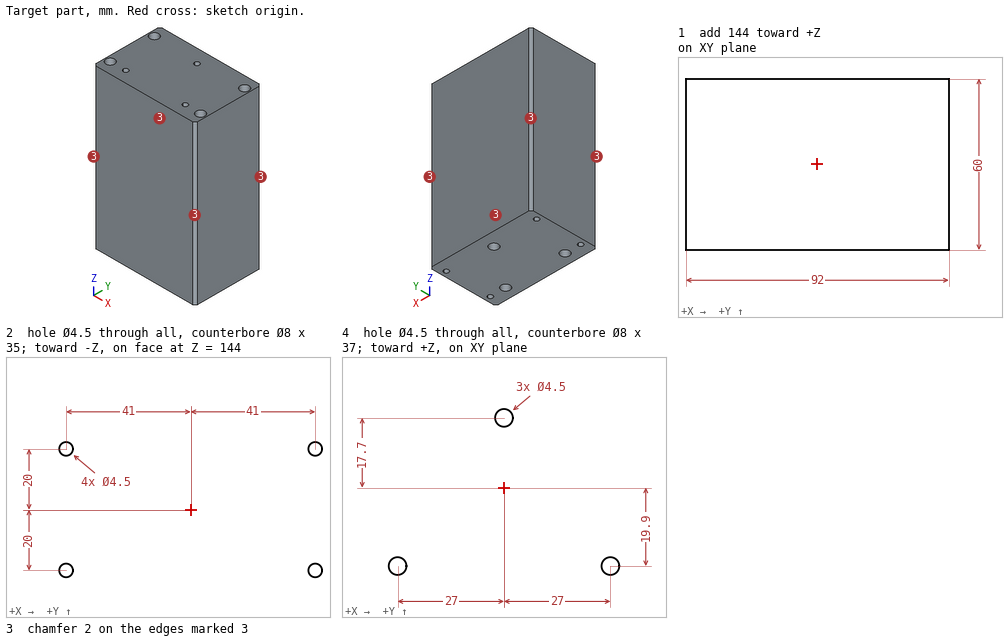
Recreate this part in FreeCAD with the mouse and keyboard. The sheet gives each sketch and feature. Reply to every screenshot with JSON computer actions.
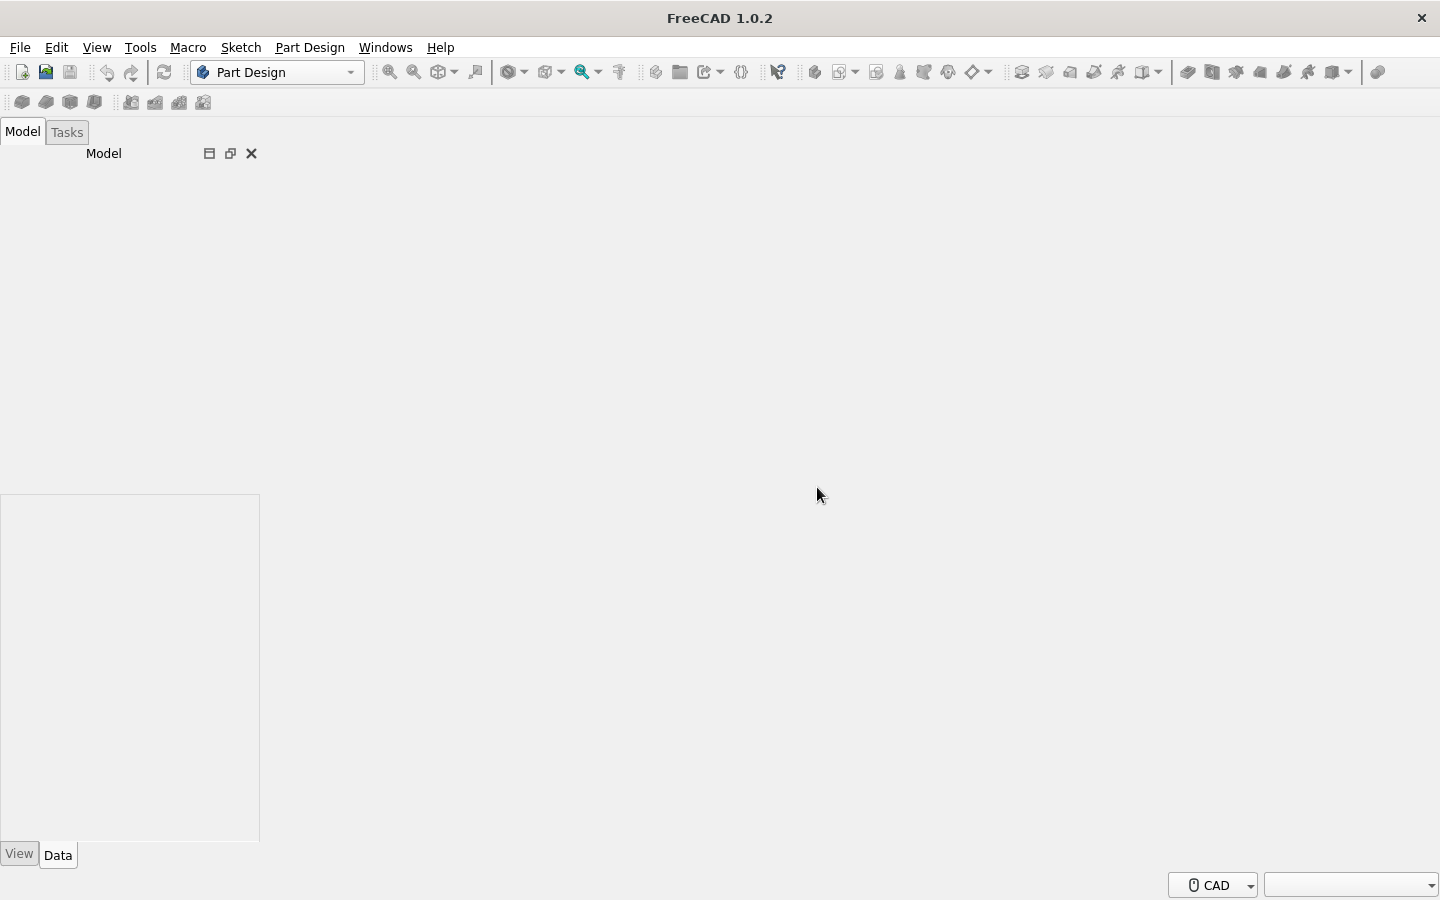
{"action": "left_click", "coordinate": [22, 72]}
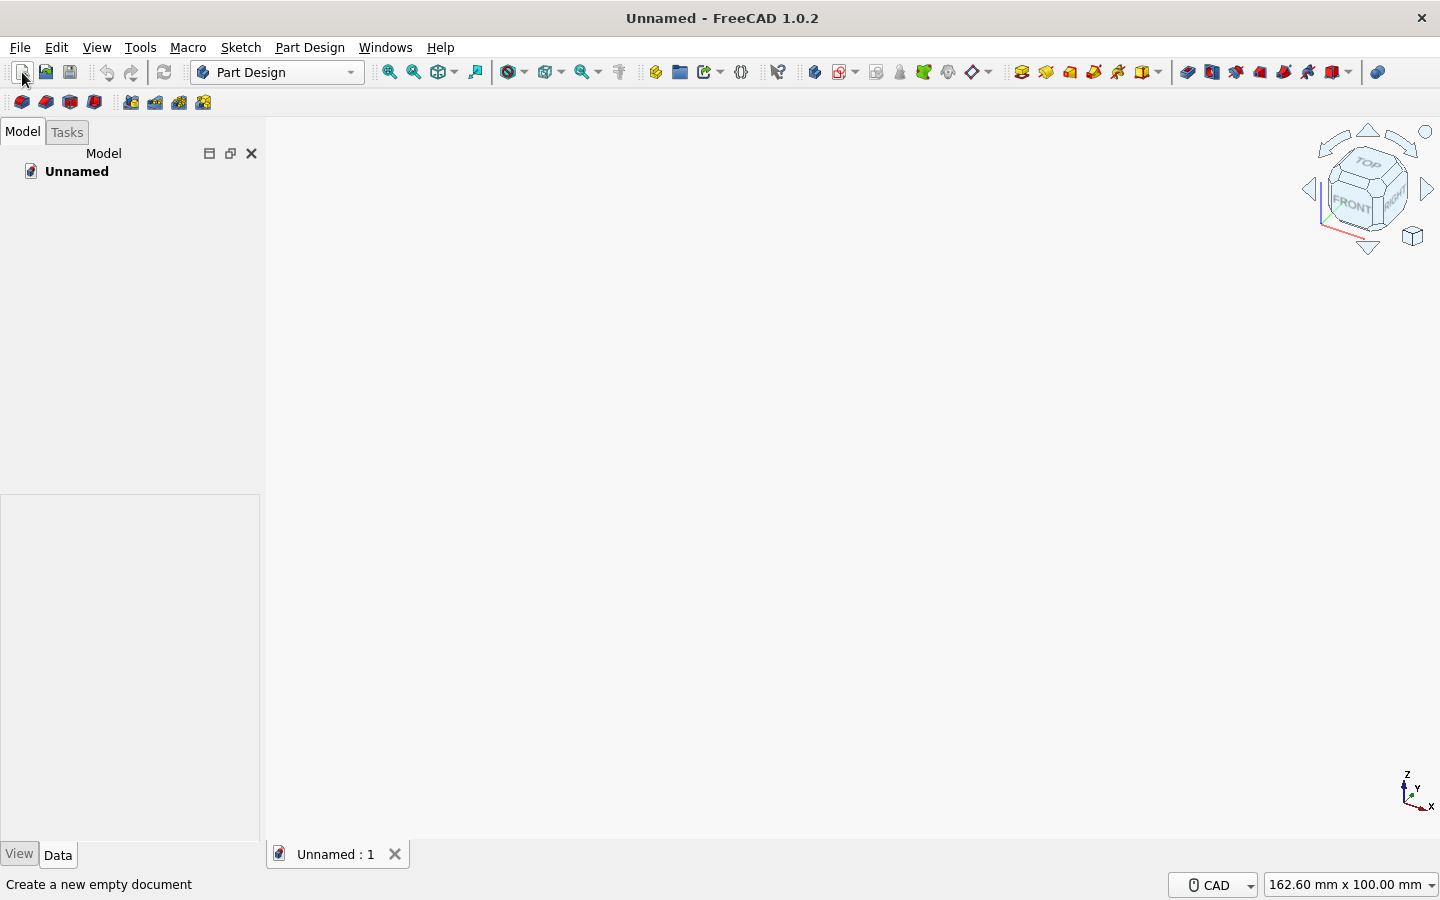
{"action": "left_click", "coordinate": [840, 72]}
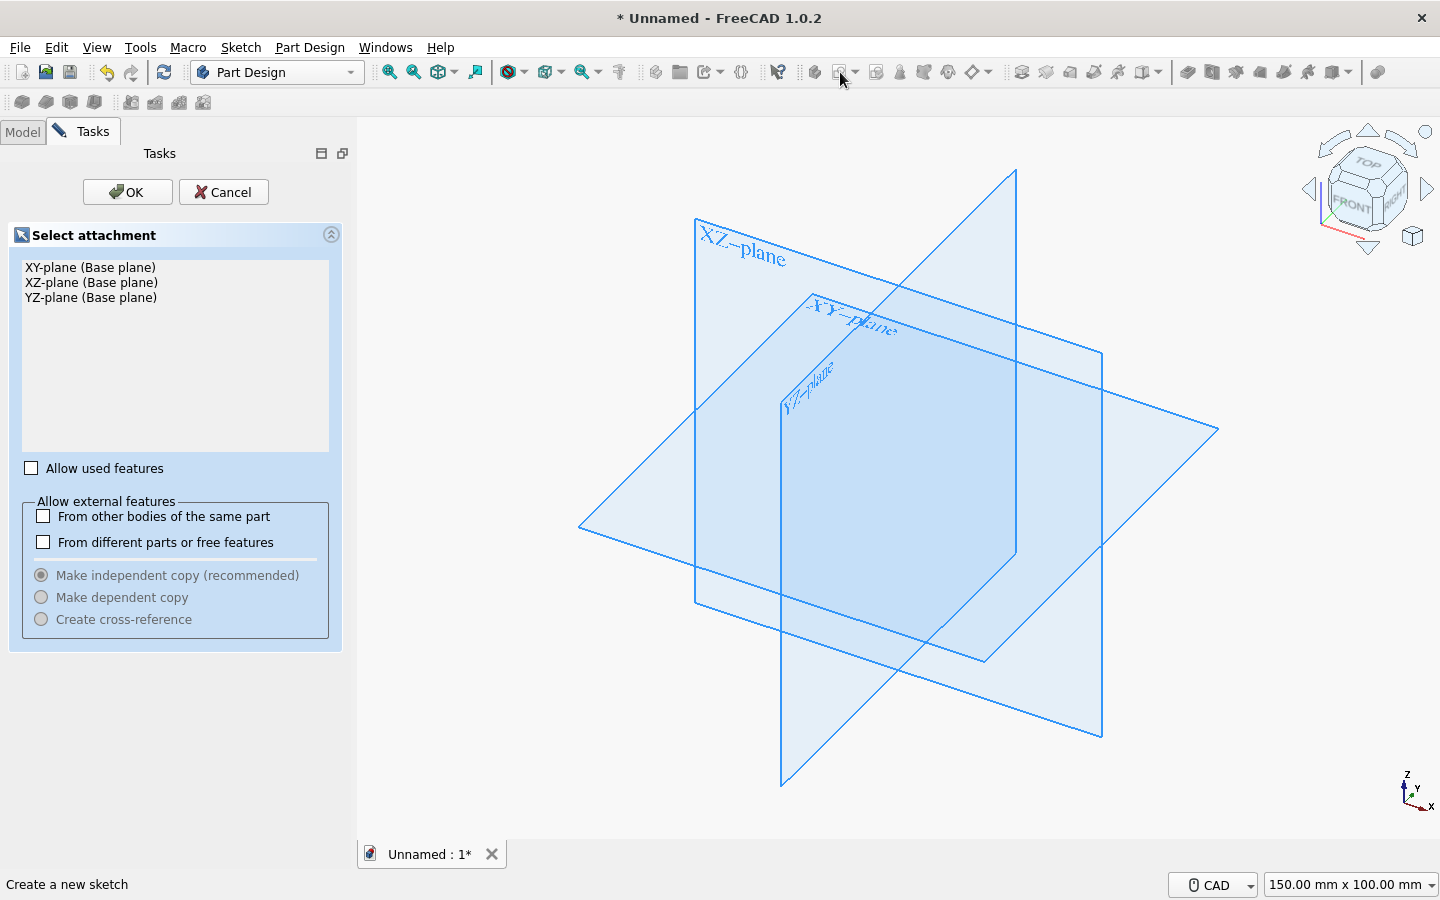
{"action": "left_click", "coordinate": [82, 268]}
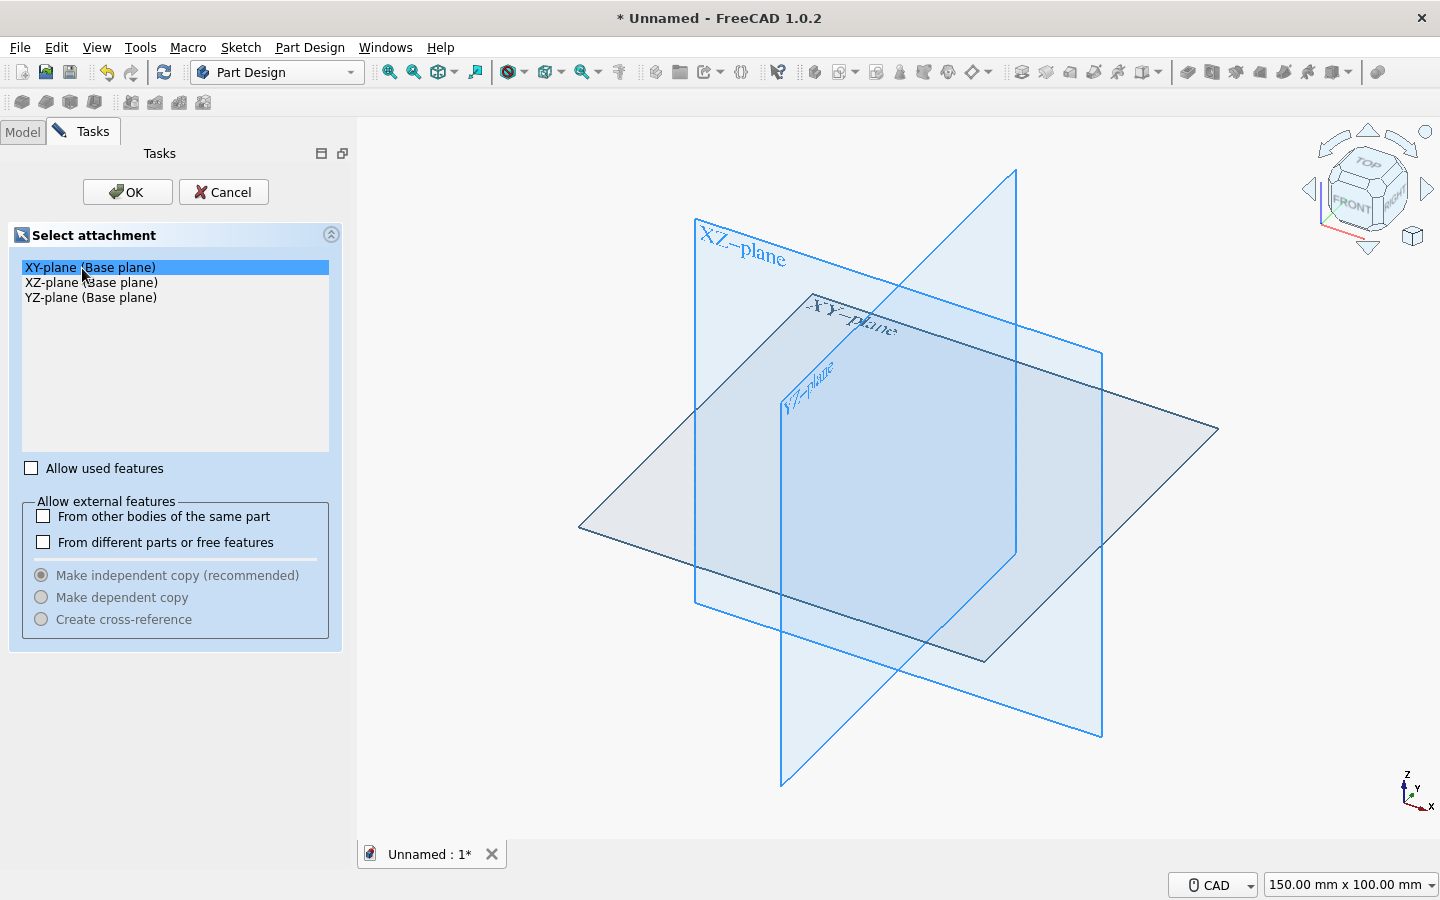
{"action": "left_click", "coordinate": [128, 192]}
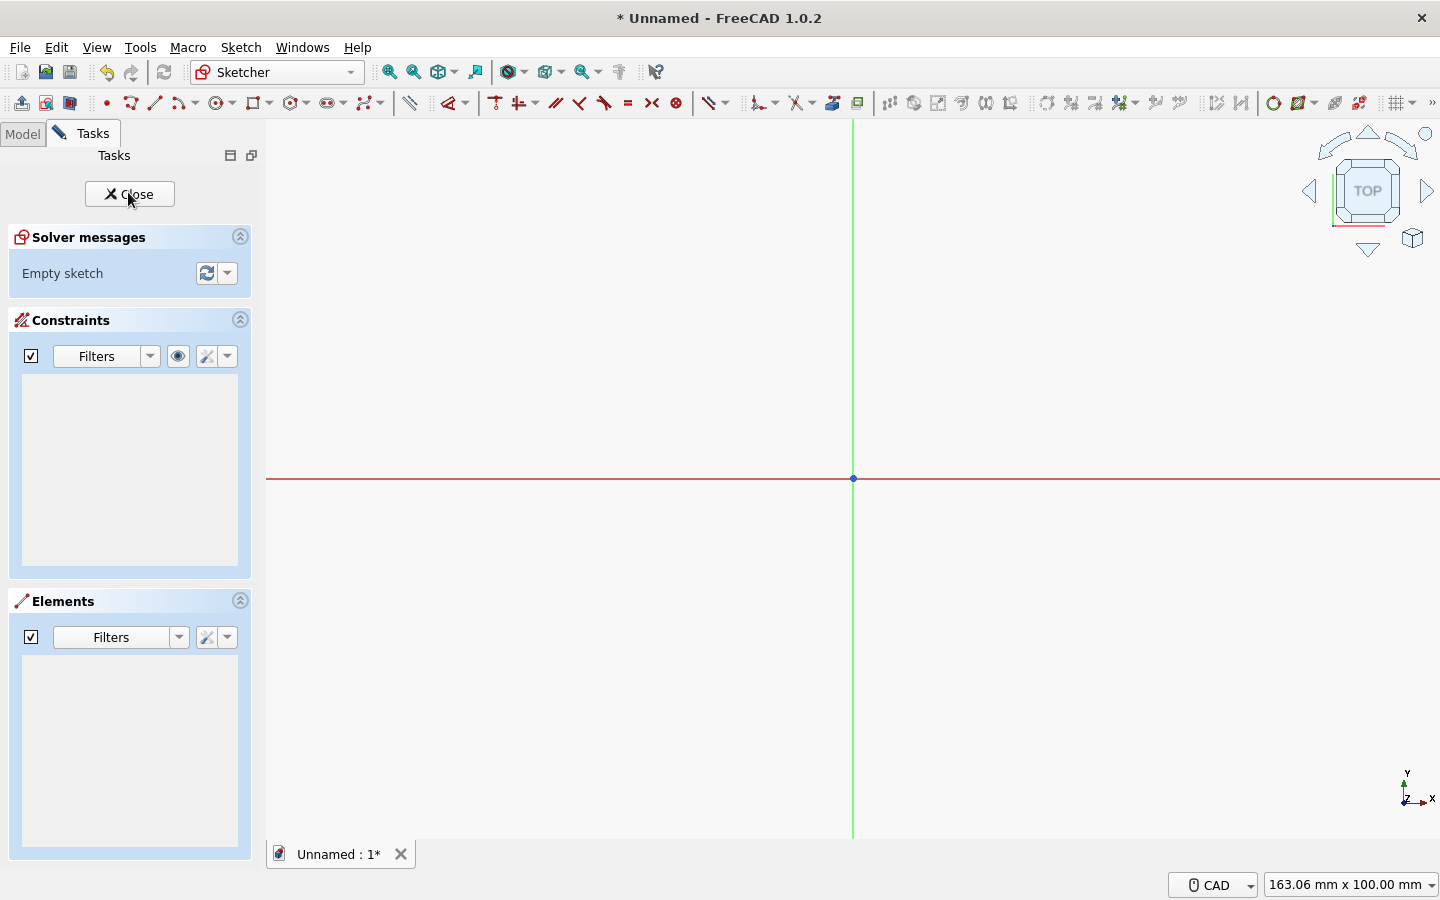
{"action": "left_click", "coordinate": [272, 104]}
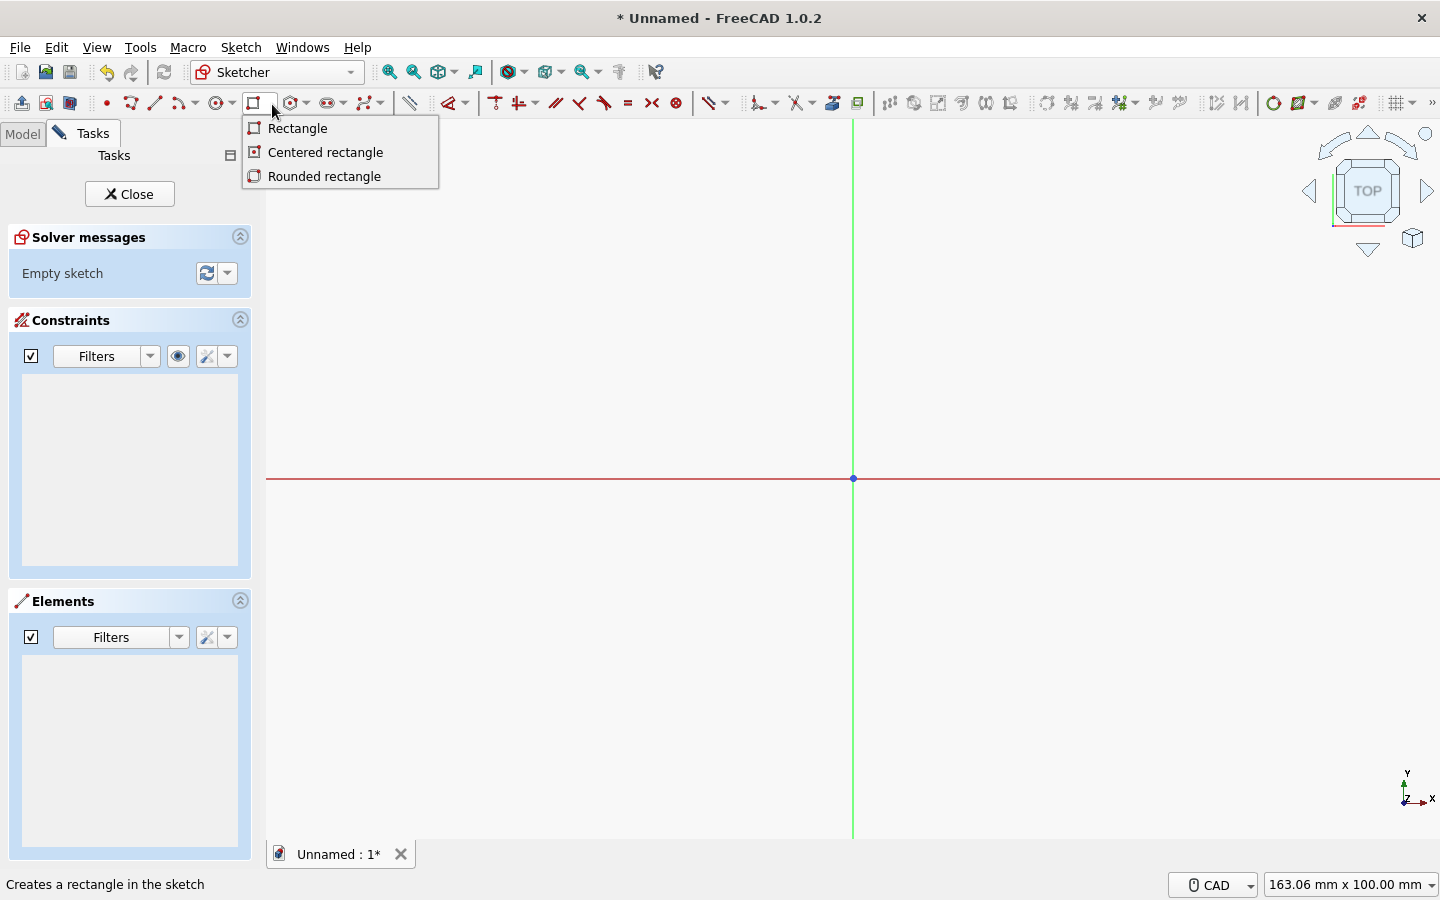
{"action": "left_click", "coordinate": [340, 152]}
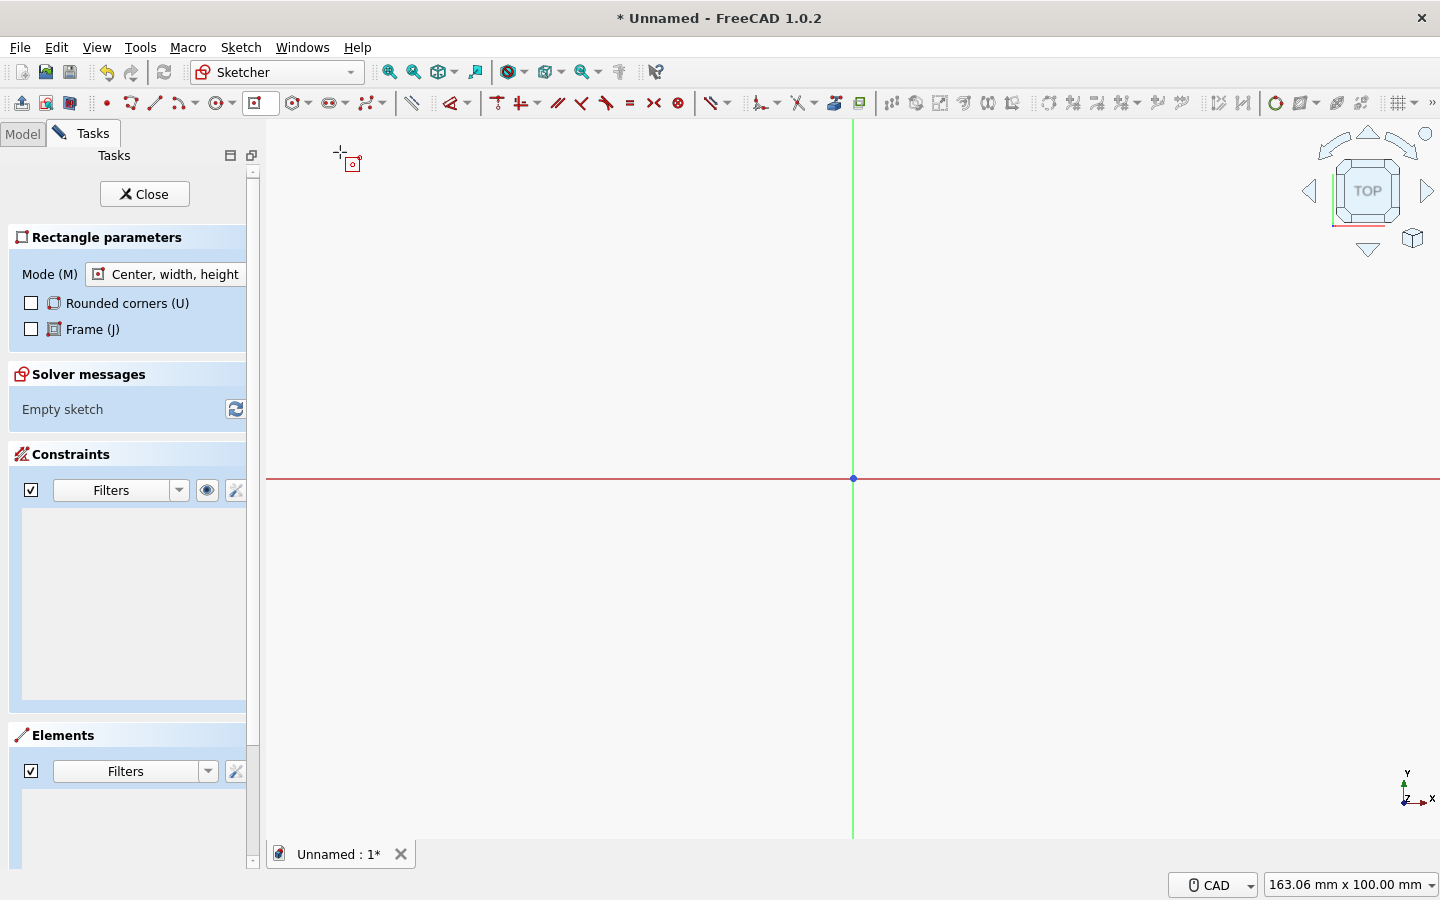
{"action": "left_click", "coordinate": [853, 479]}
{"action": "left_click", "coordinate": [1184, 263]}
{"action": "key", "text": "Escape"}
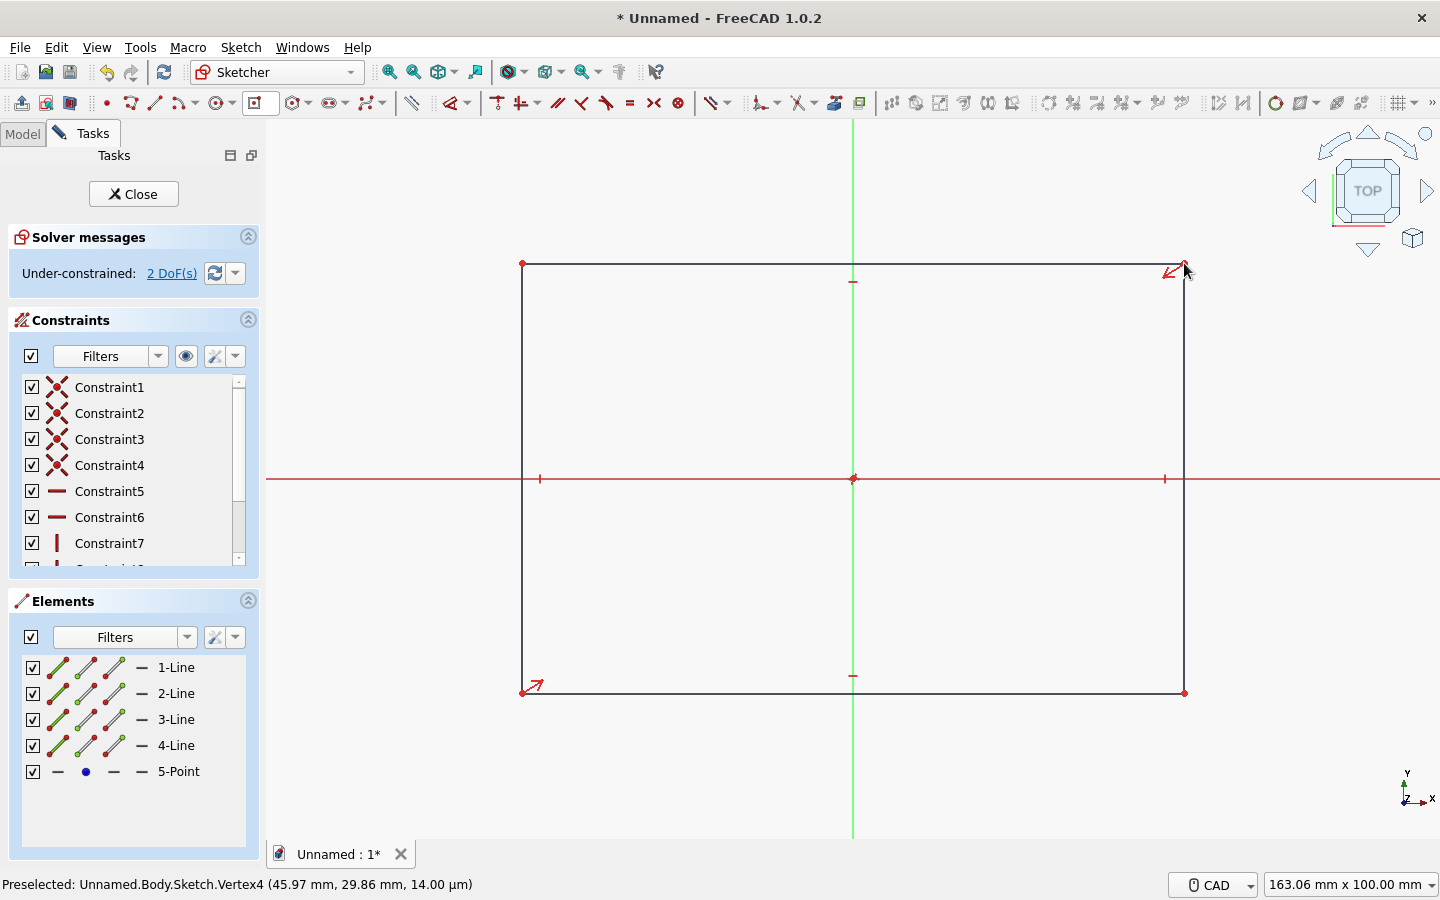
{"action": "left_click", "coordinate": [450, 104]}